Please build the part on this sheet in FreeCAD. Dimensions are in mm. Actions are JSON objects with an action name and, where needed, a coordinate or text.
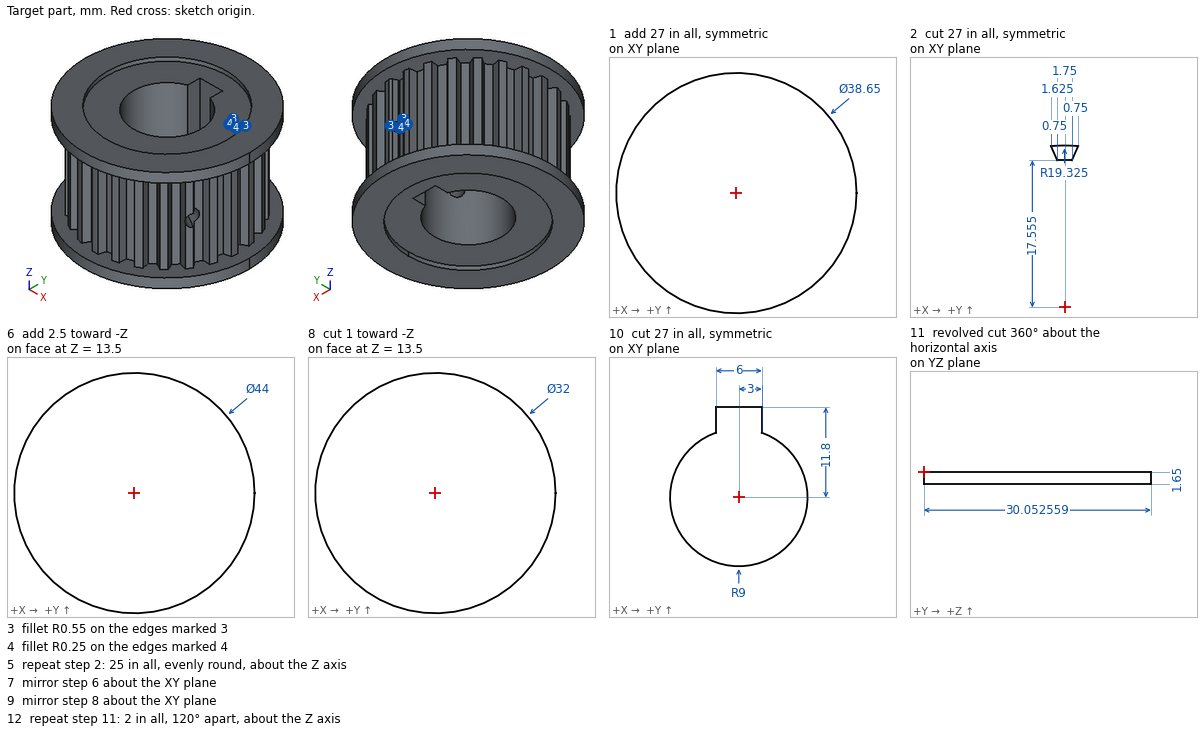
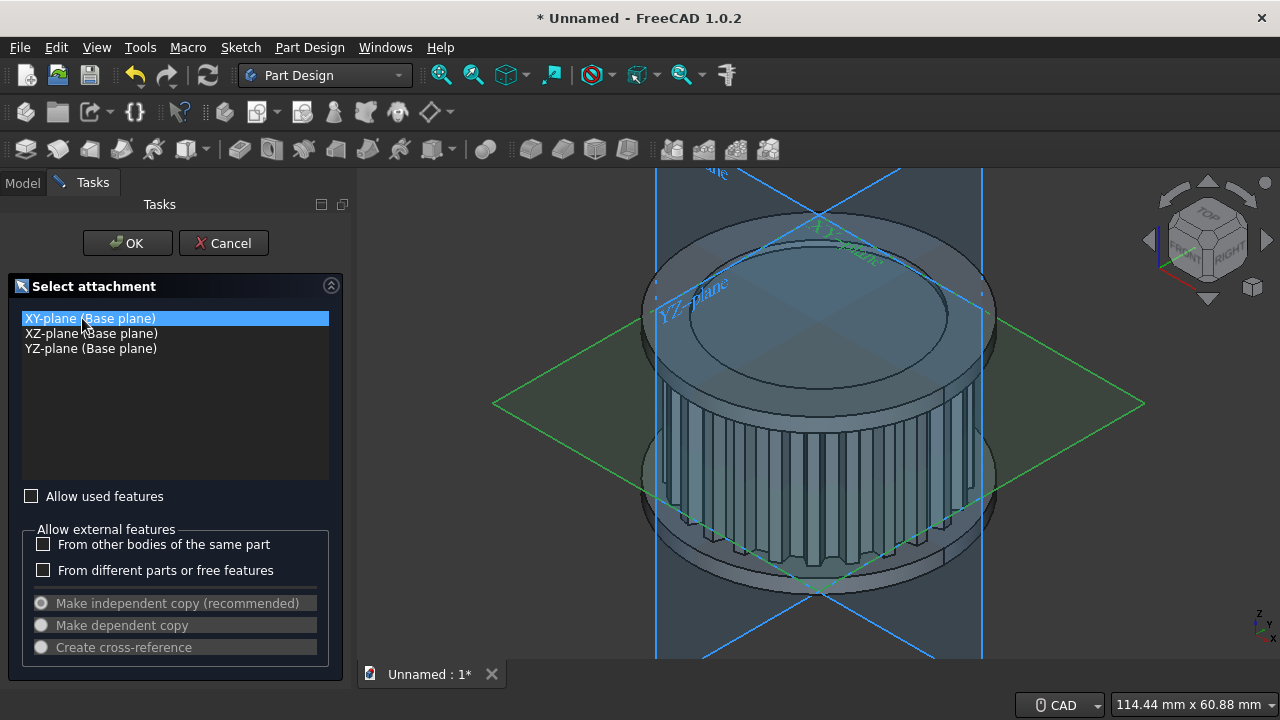
{"action": "left_click", "coordinate": [128, 243]}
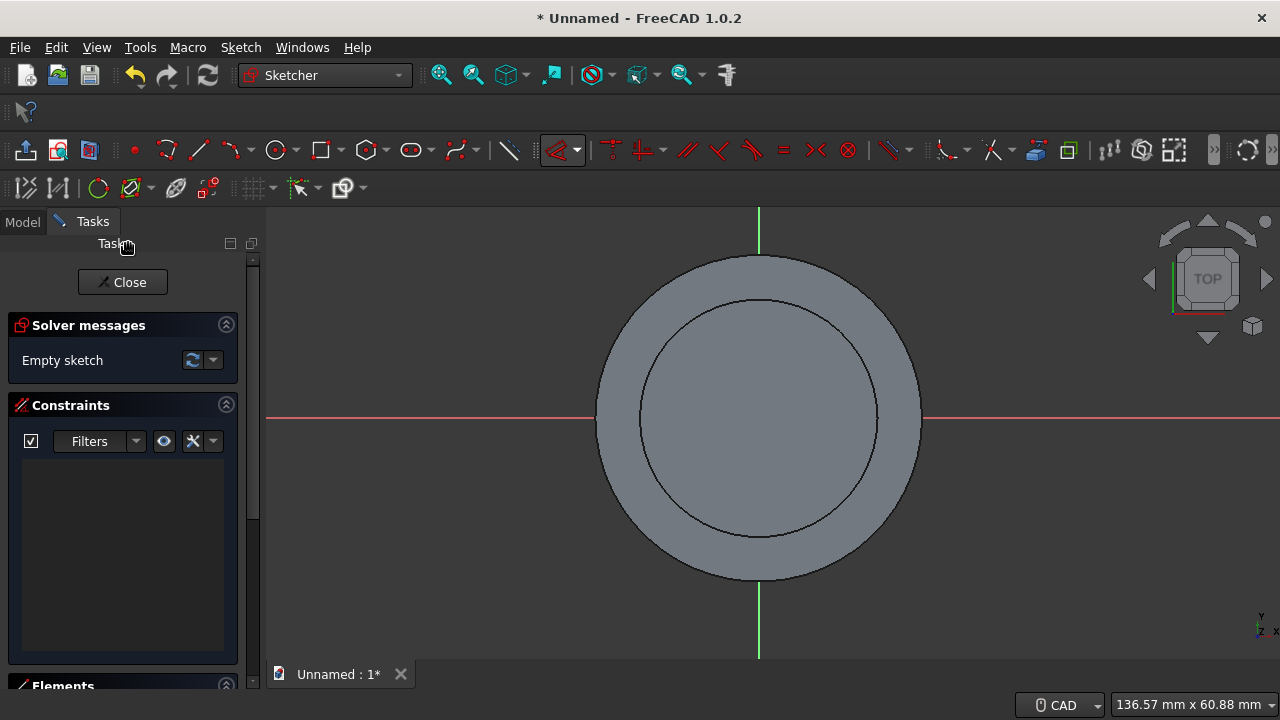
{"action": "left_click", "coordinate": [90, 150]}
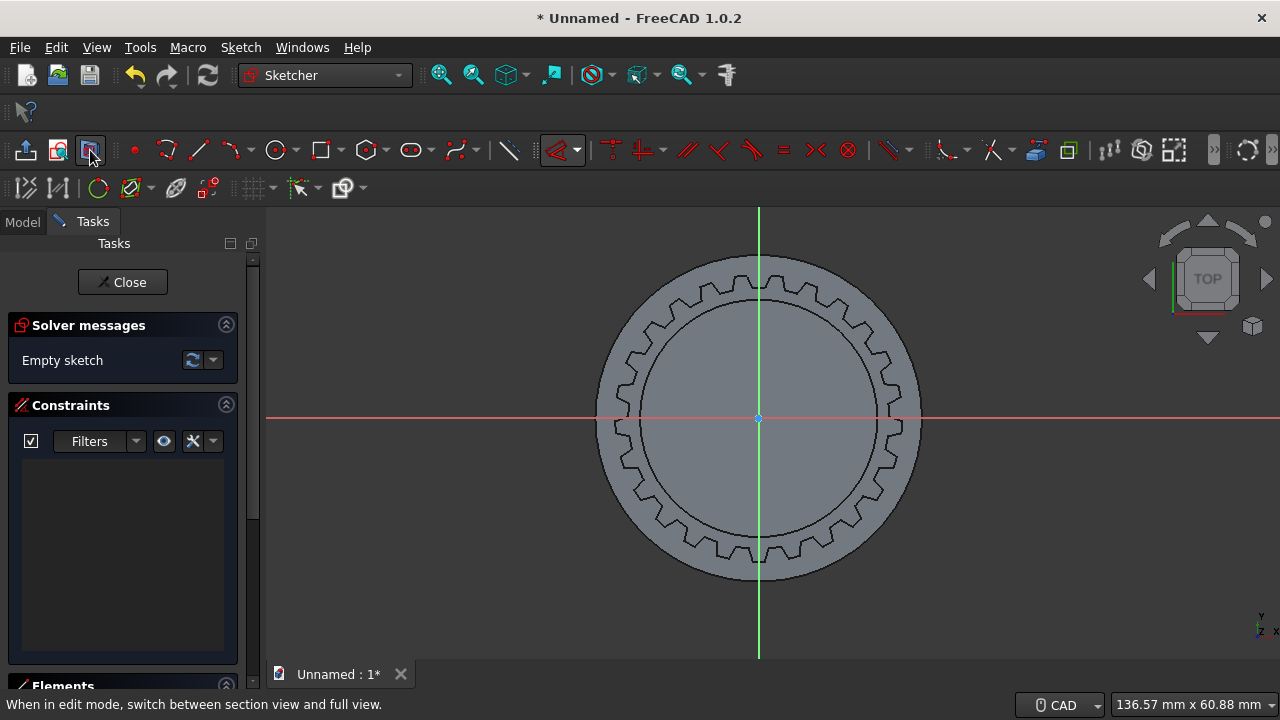
{"action": "scroll", "coordinate": [825, 378], "scroll_direction": "up", "scroll_amount": 3}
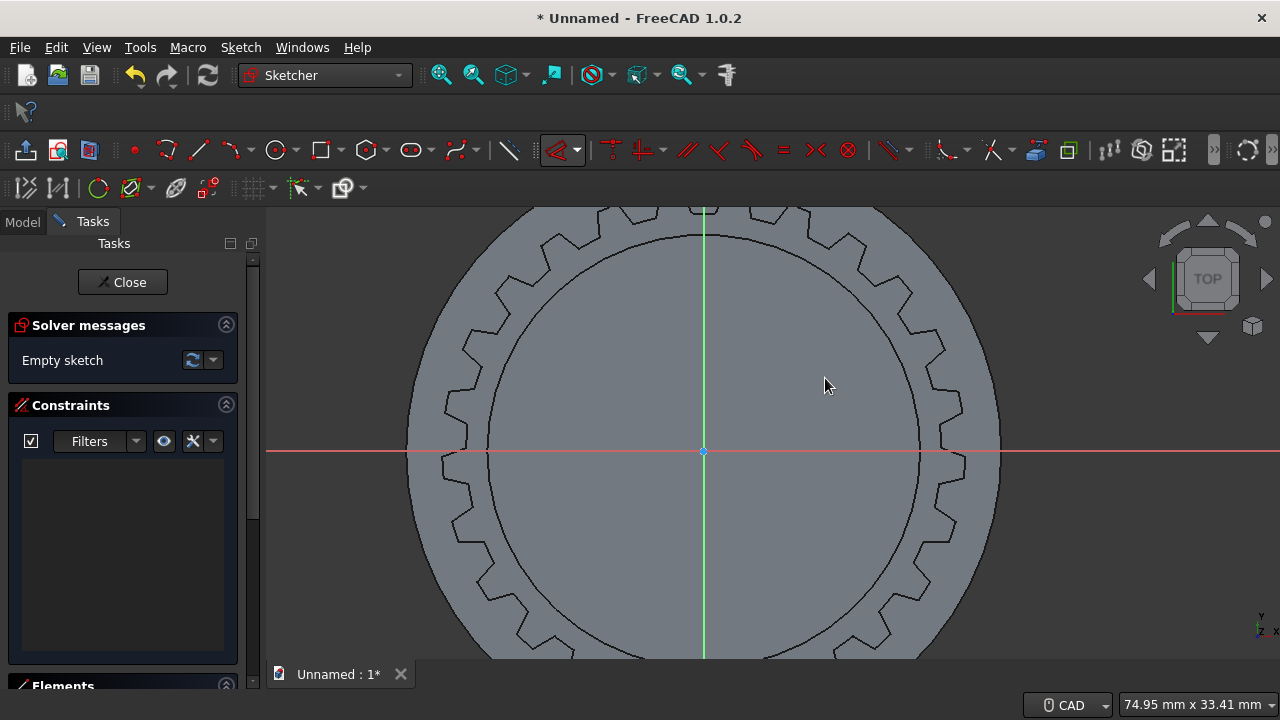
{"action": "left_click", "coordinate": [168, 150]}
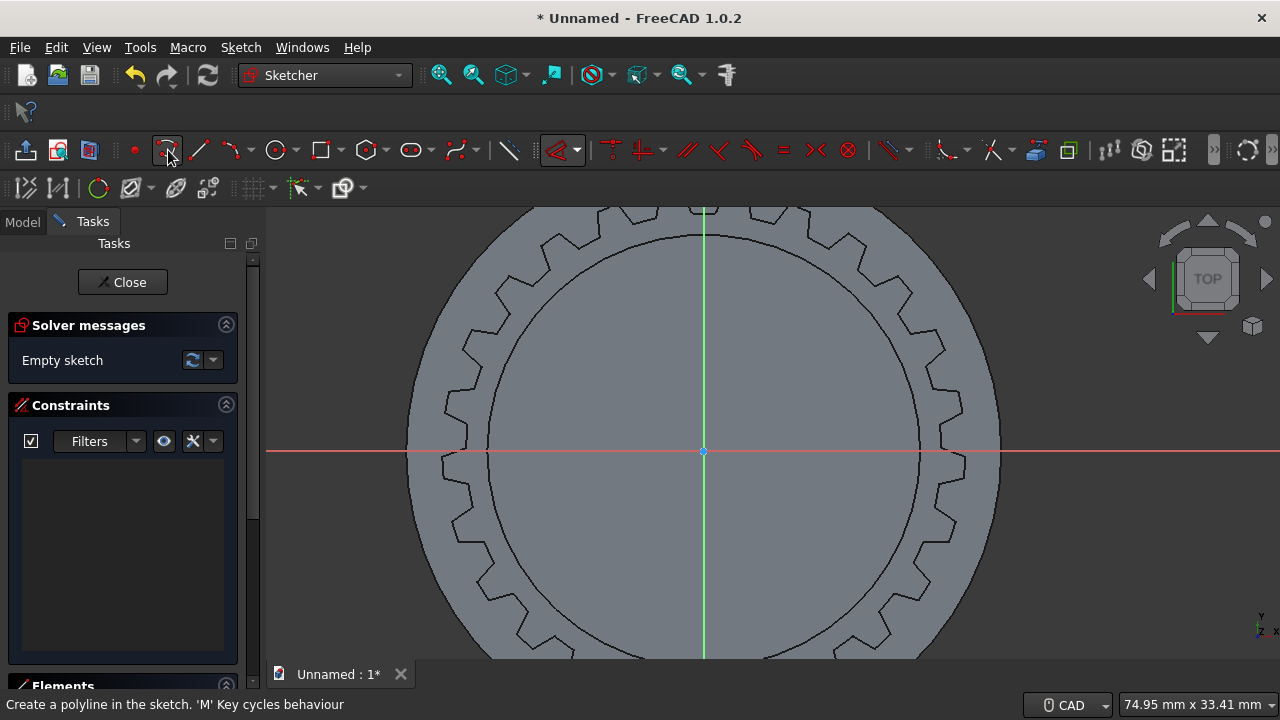
{"action": "left_click", "coordinate": [744, 336]}
{"action": "left_click", "coordinate": [744, 292]}
{"action": "left_click", "coordinate": [663, 292]}
{"action": "left_click", "coordinate": [663, 336]}
{"action": "right_click", "coordinate": [663, 336]}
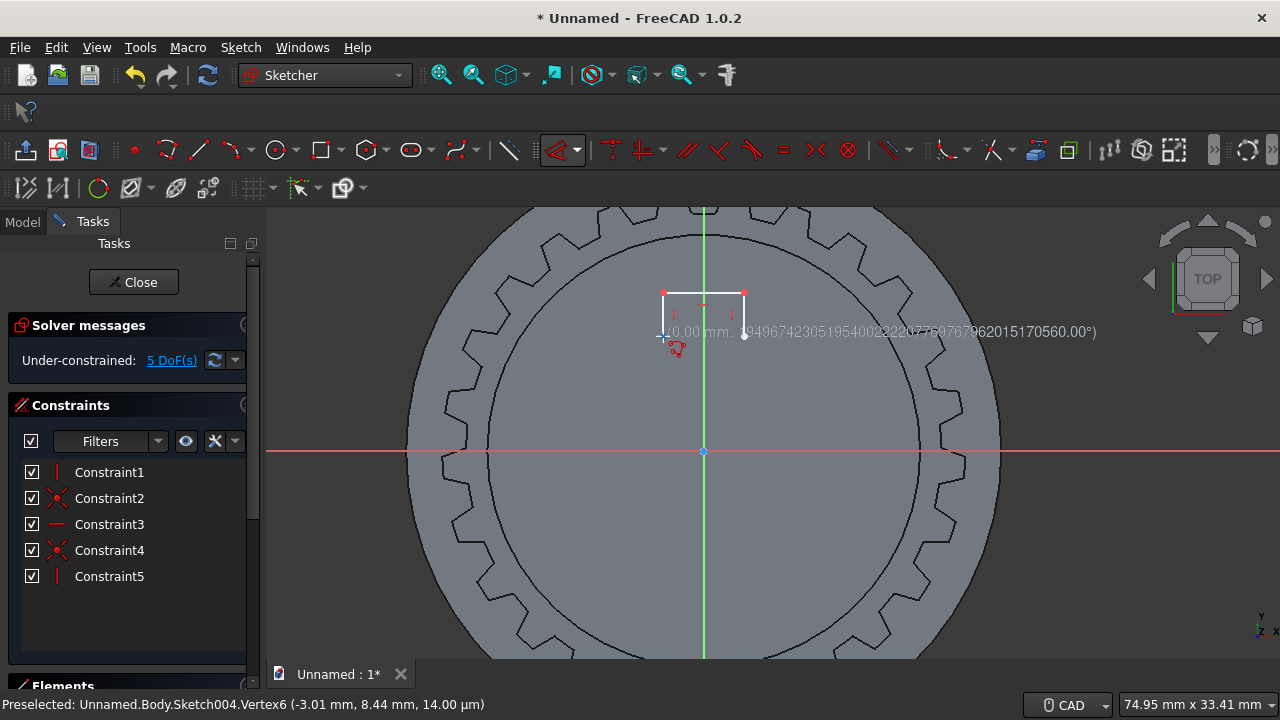
{"action": "left_click", "coordinate": [232, 150]}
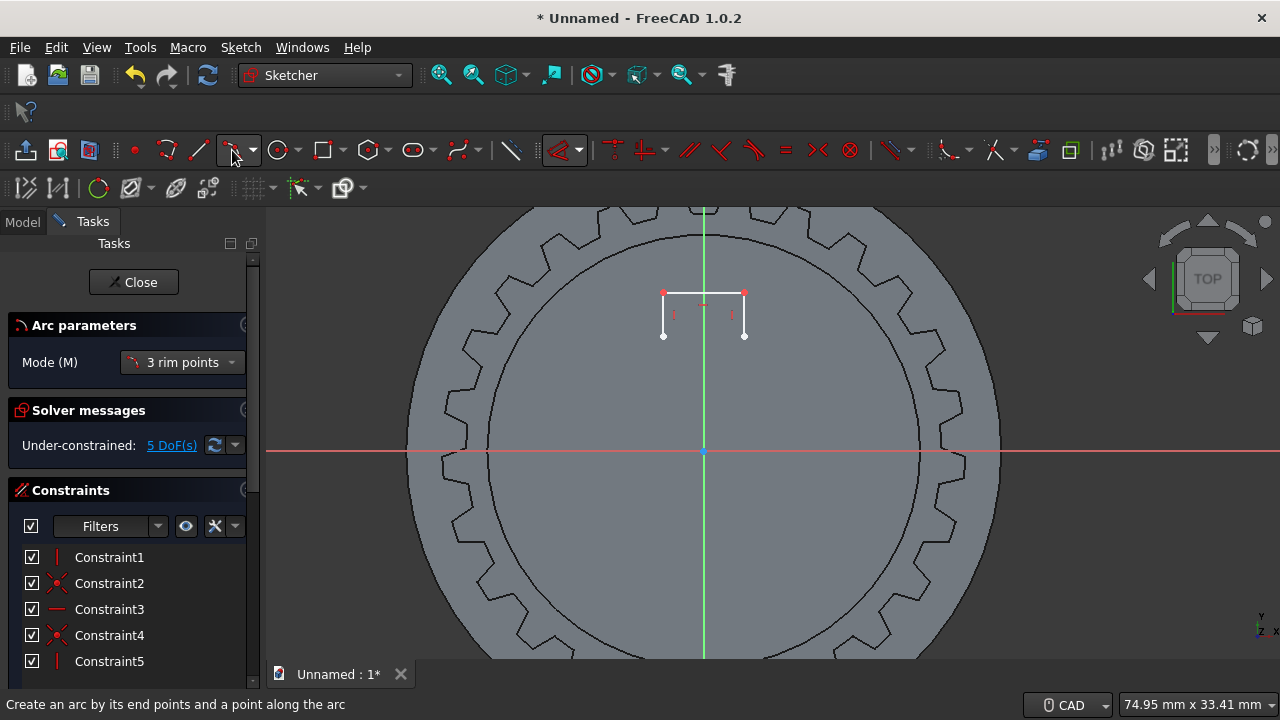
{"action": "left_click", "coordinate": [663, 337]}
{"action": "left_click", "coordinate": [744, 337]}
{"action": "left_click", "coordinate": [639, 554]}
{"action": "key", "text": "Escape"}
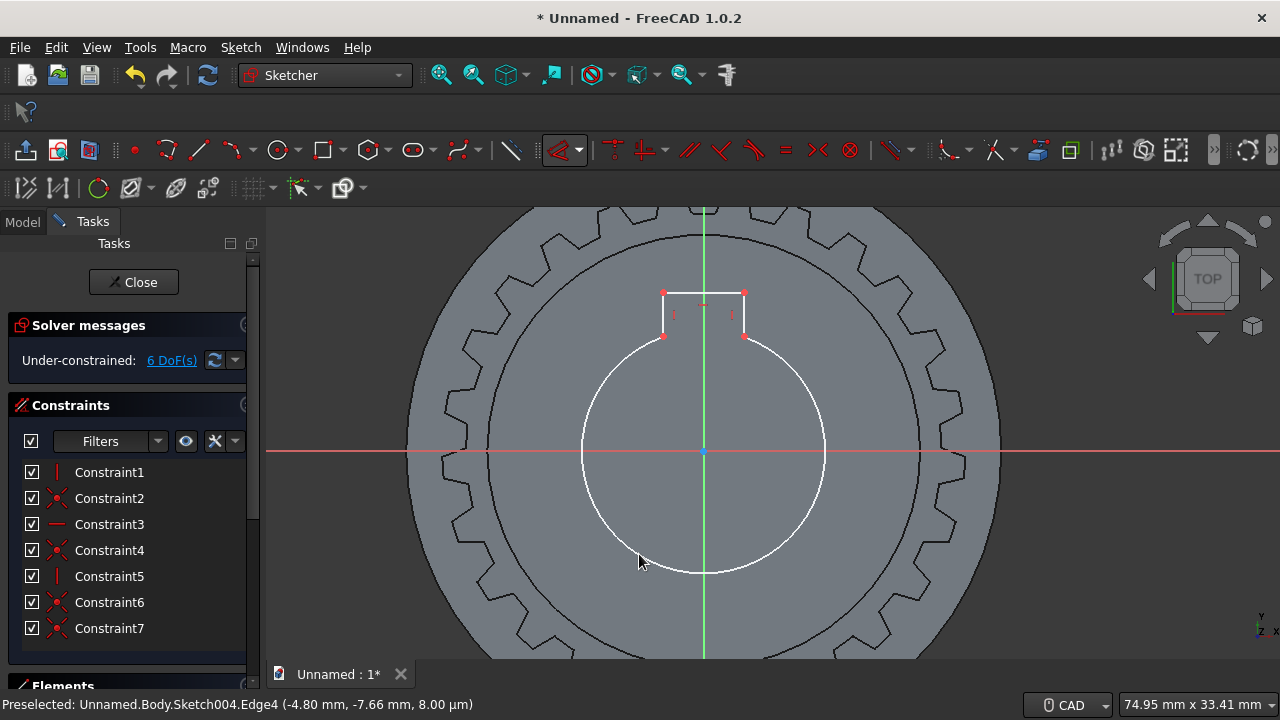
{"action": "left_click_drag", "start_coordinate": [693, 441], "coordinate": [714, 462]}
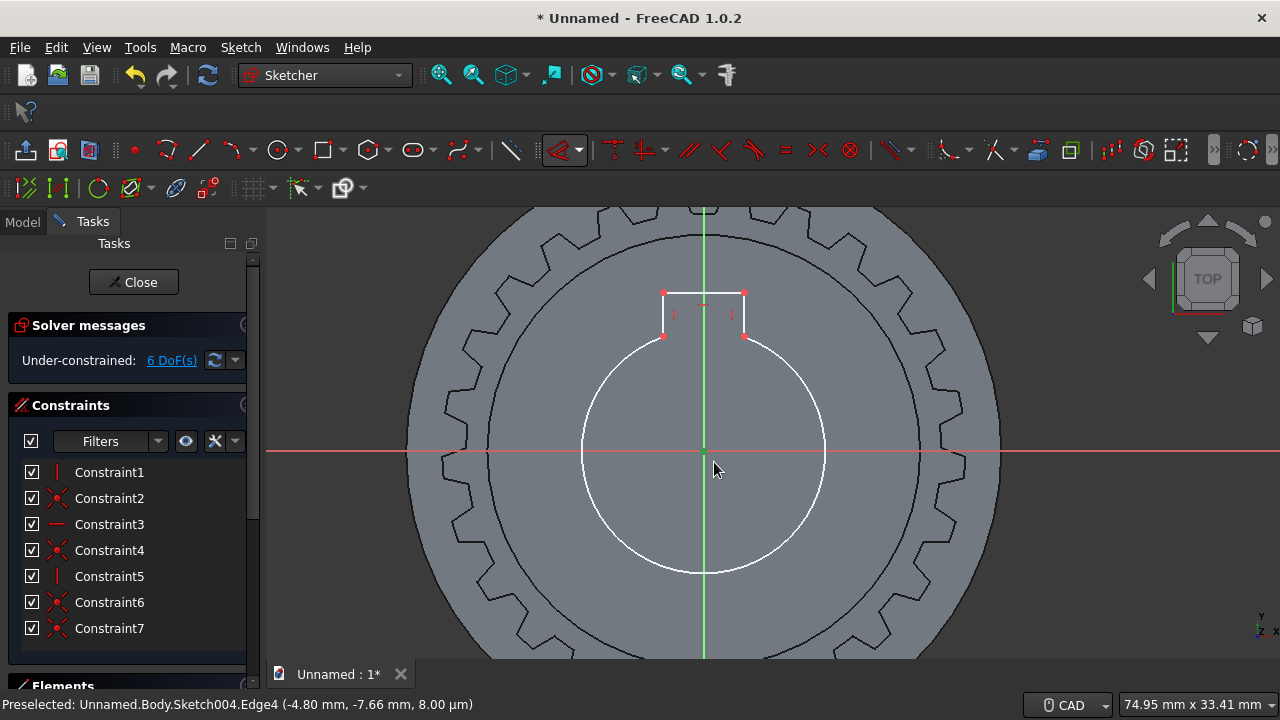
{"action": "left_click", "coordinate": [614, 150]}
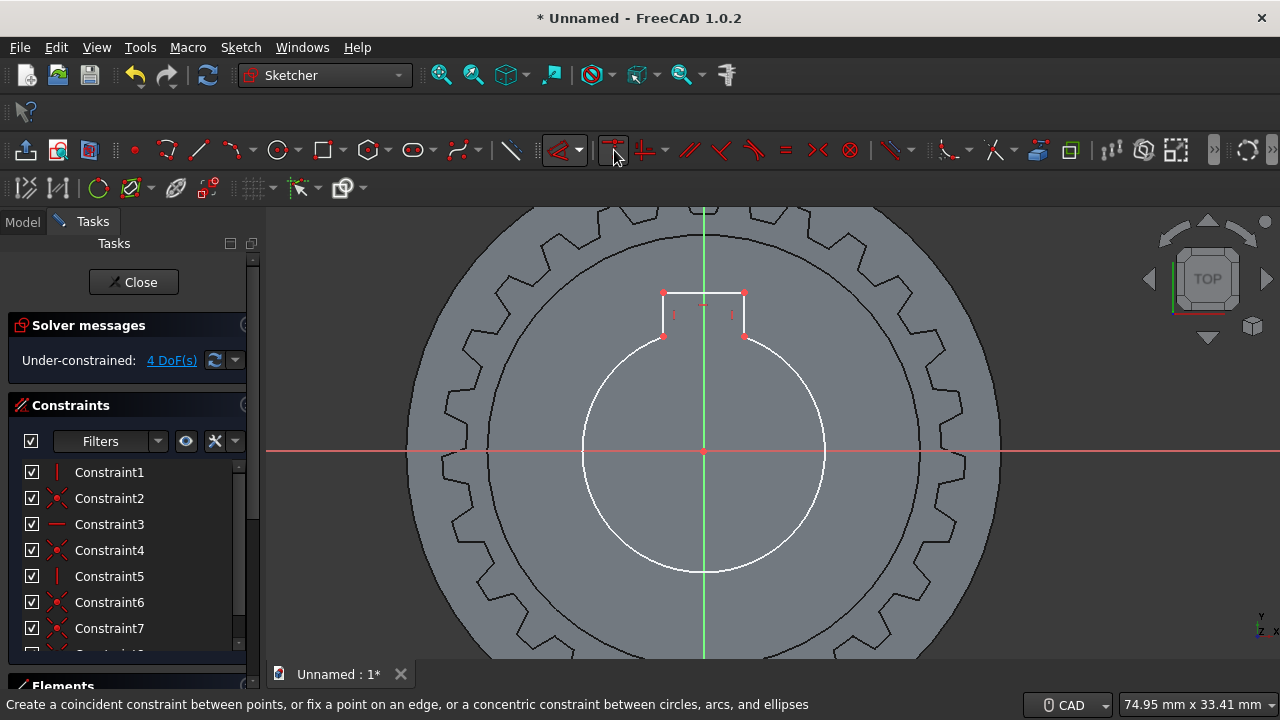
{"action": "left_click", "coordinate": [595, 504]}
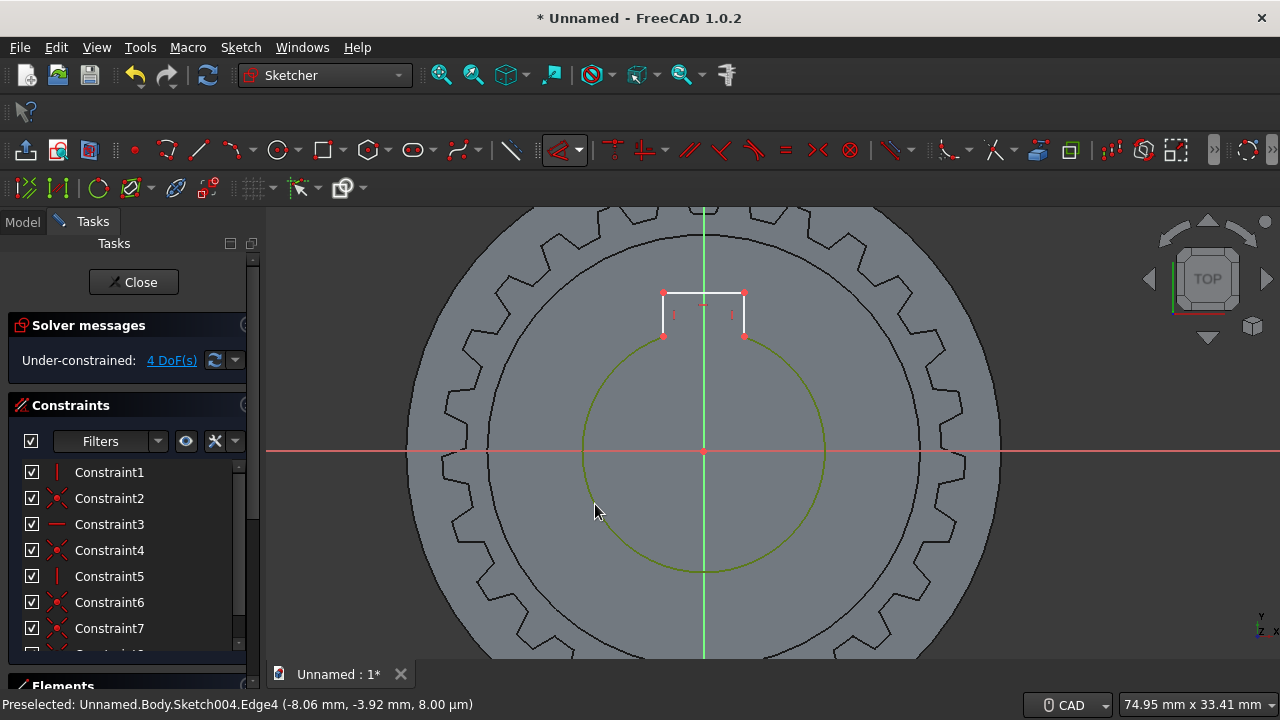
{"action": "key", "text": "k r"}